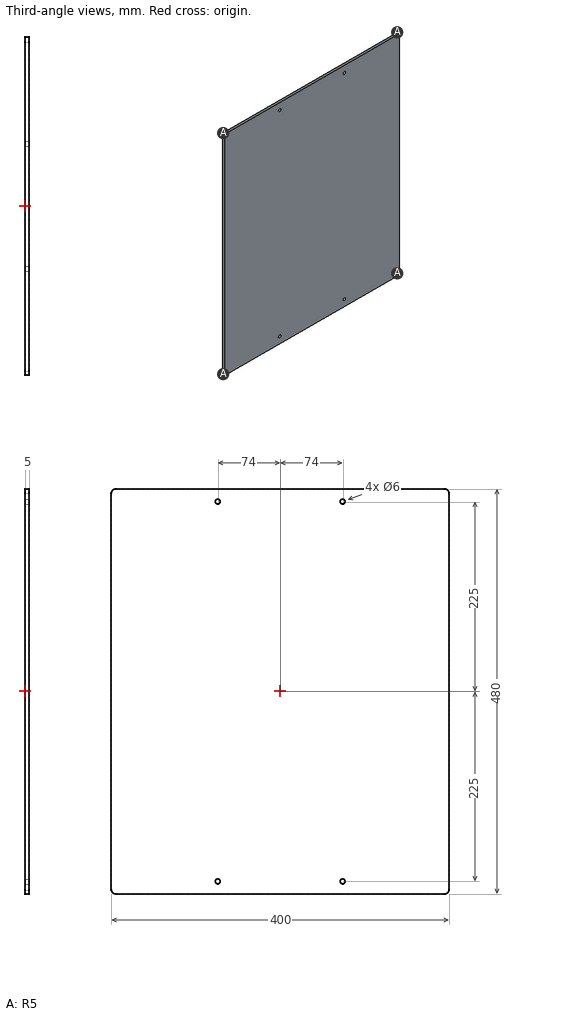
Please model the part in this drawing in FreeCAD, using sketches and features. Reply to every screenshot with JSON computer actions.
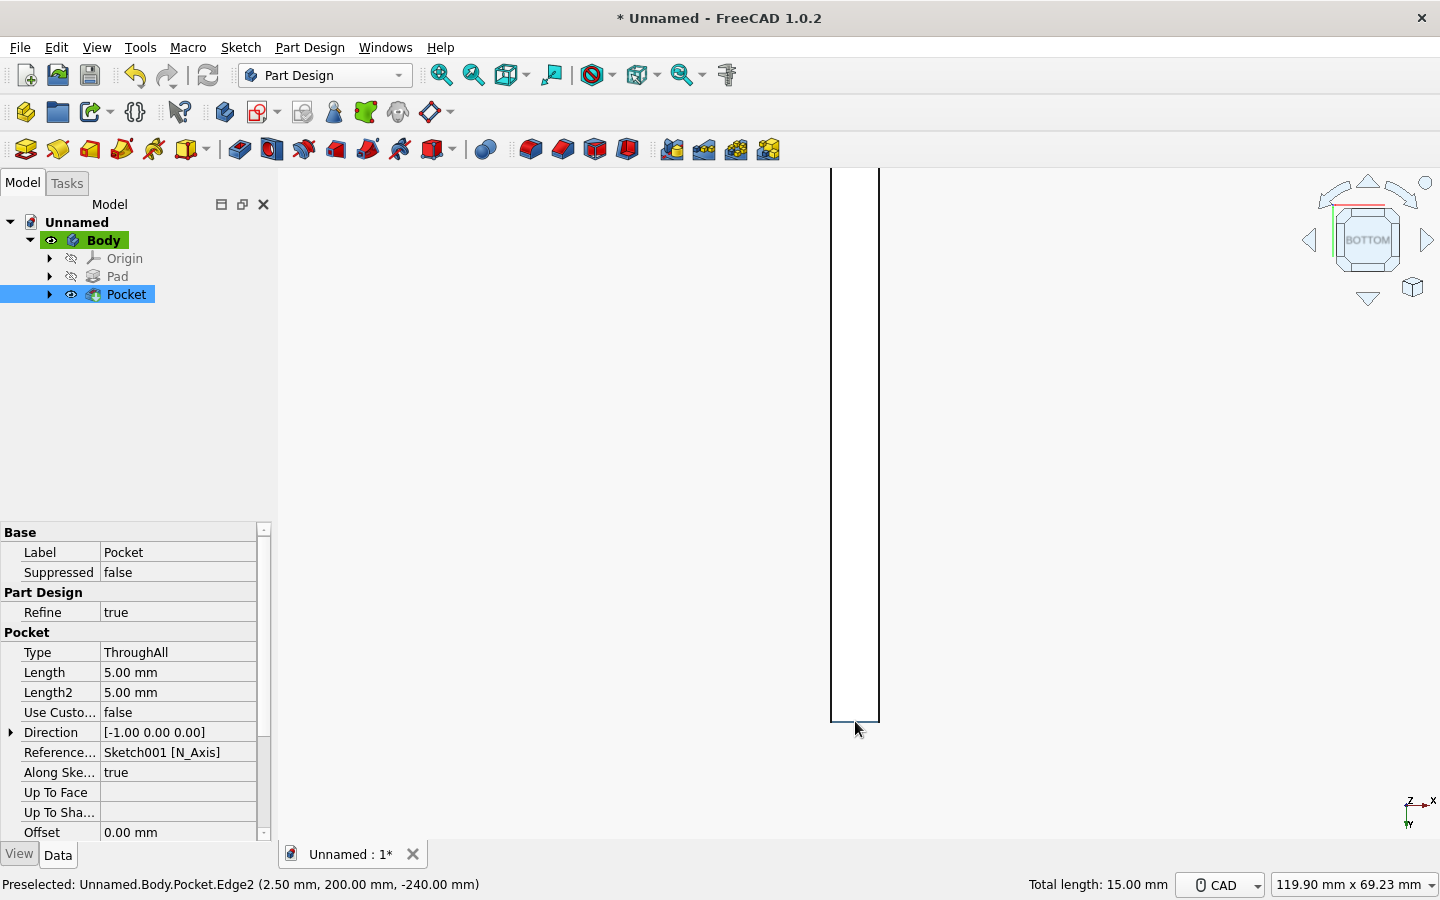
{"action": "key", "text": "v f"}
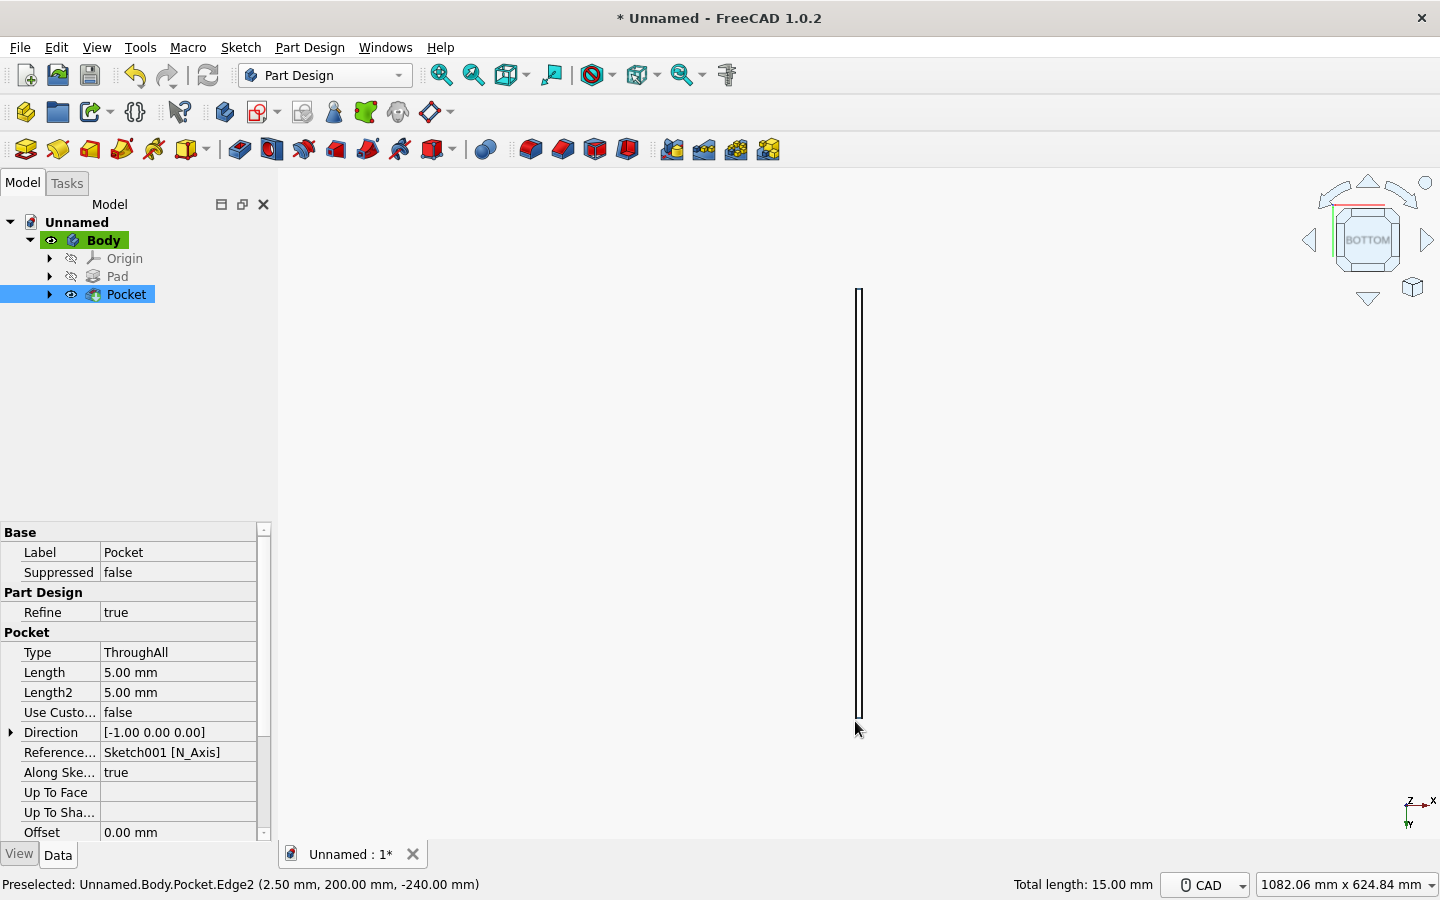
{"action": "key", "text": "4"}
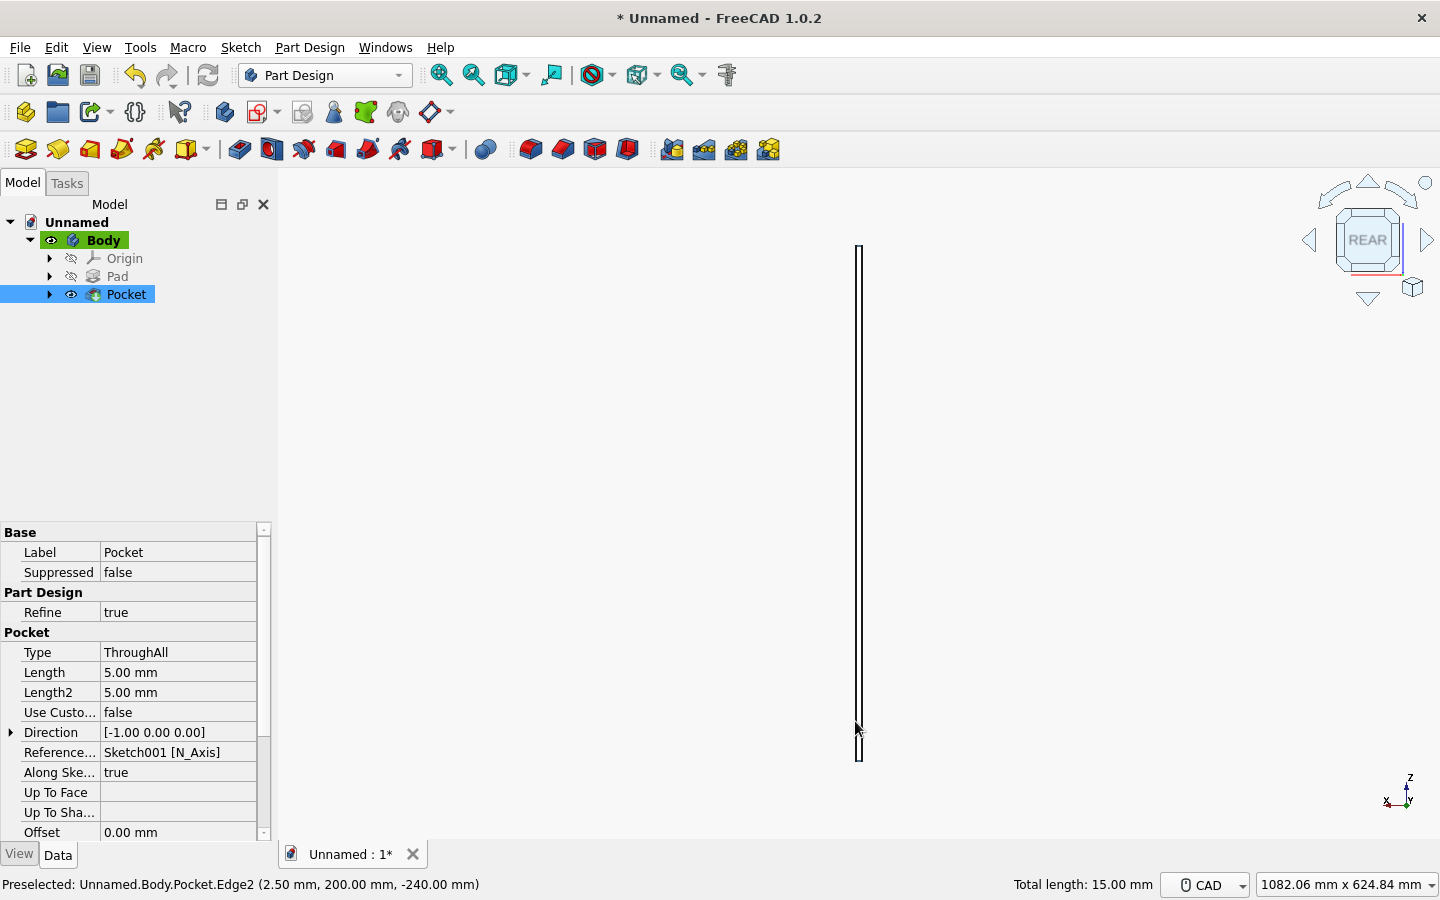
{"action": "scroll", "coordinate": [859, 245], "scroll_direction": "up", "scroll_amount": 11}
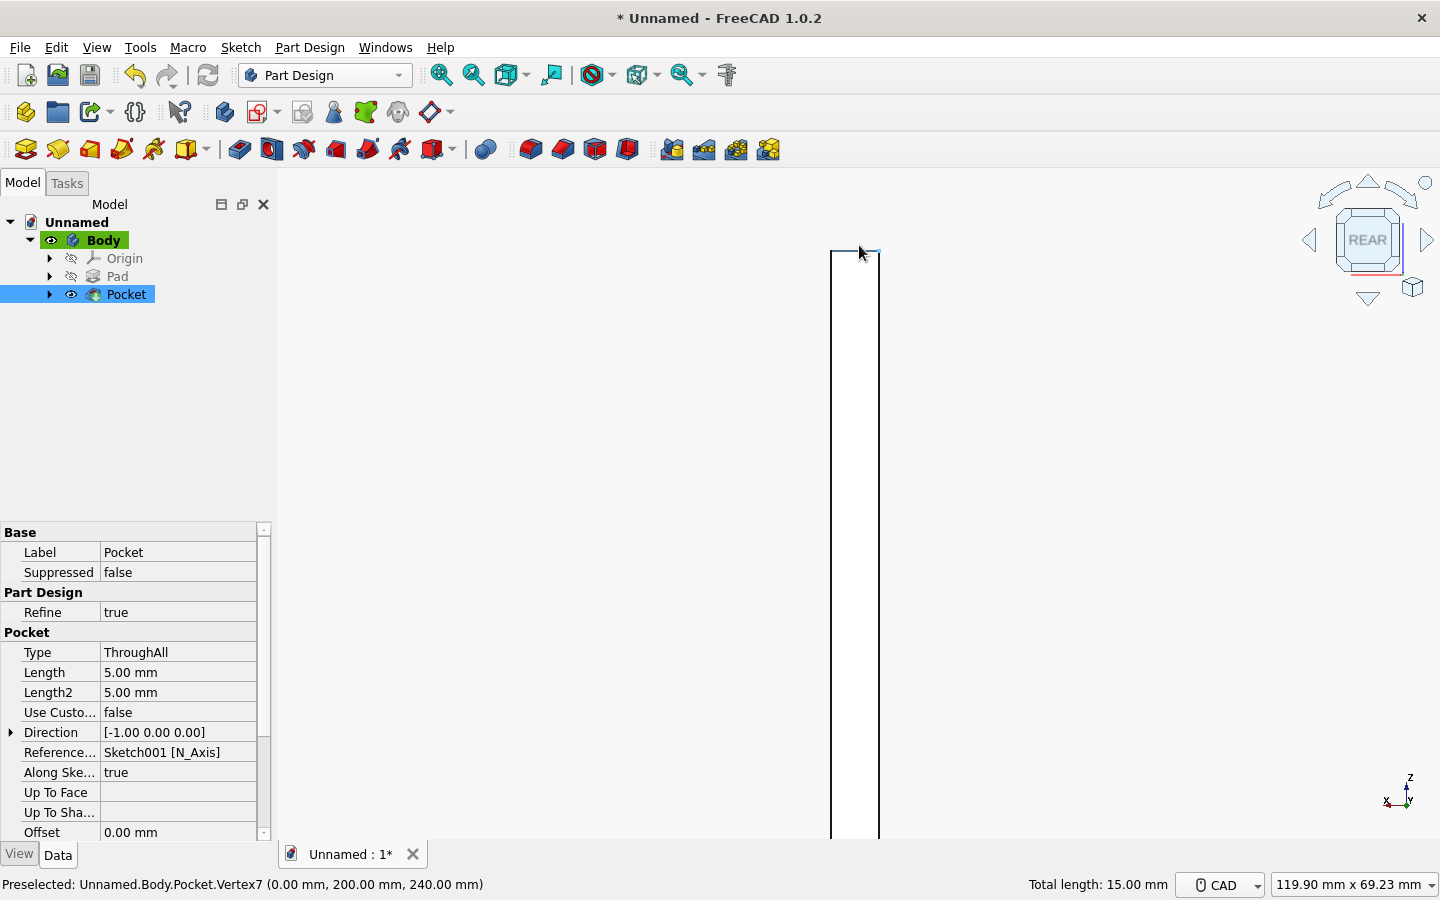
{"action": "left_click", "coordinate": [442, 76]}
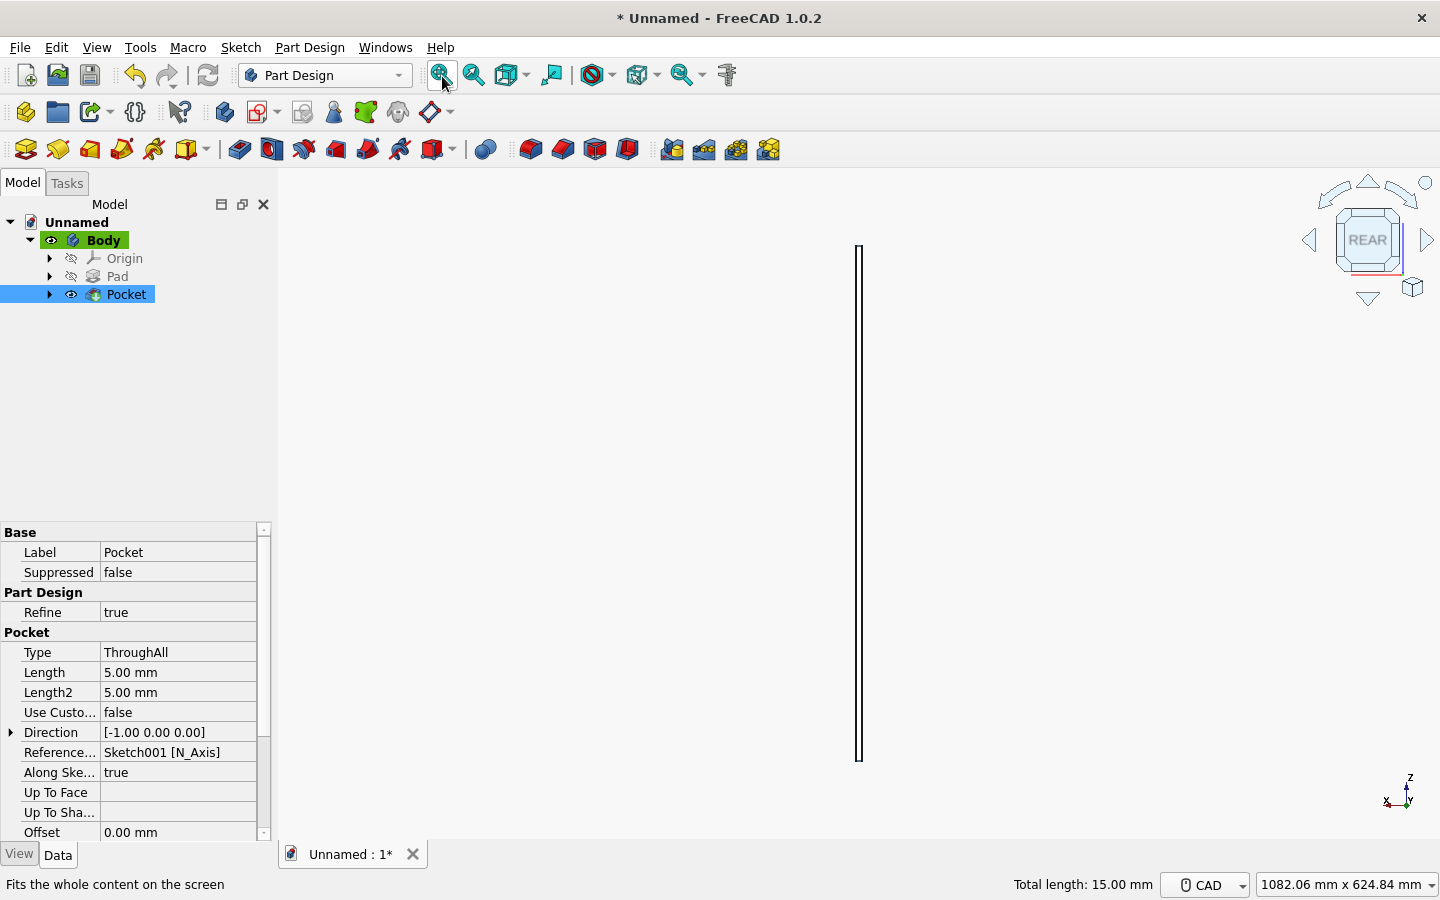
{"action": "key", "text": "6"}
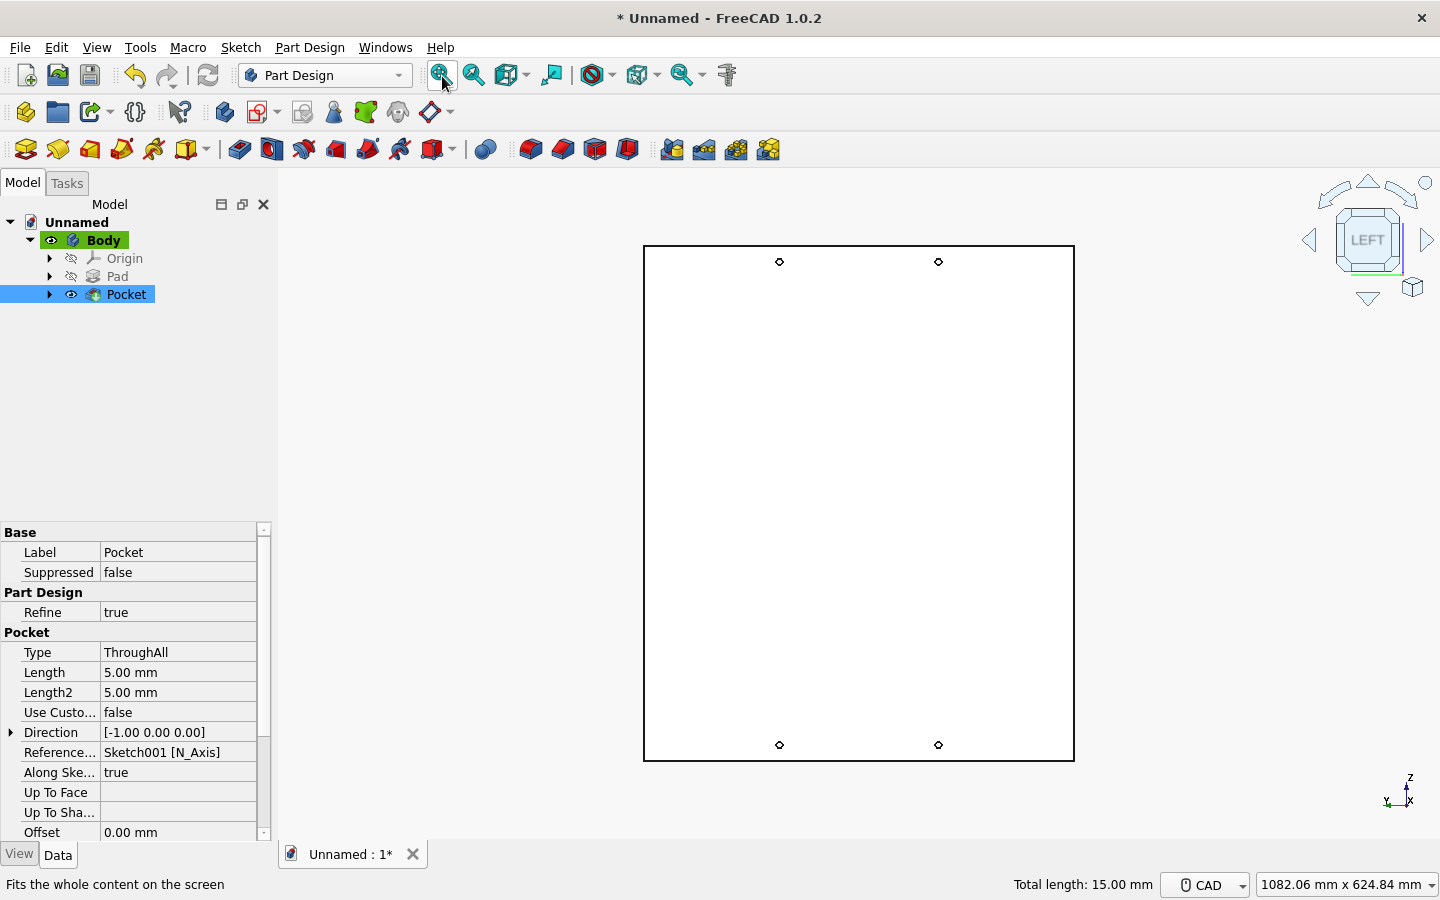
{"action": "scroll", "coordinate": [1074, 245], "scroll_direction": "up", "scroll_amount": 11}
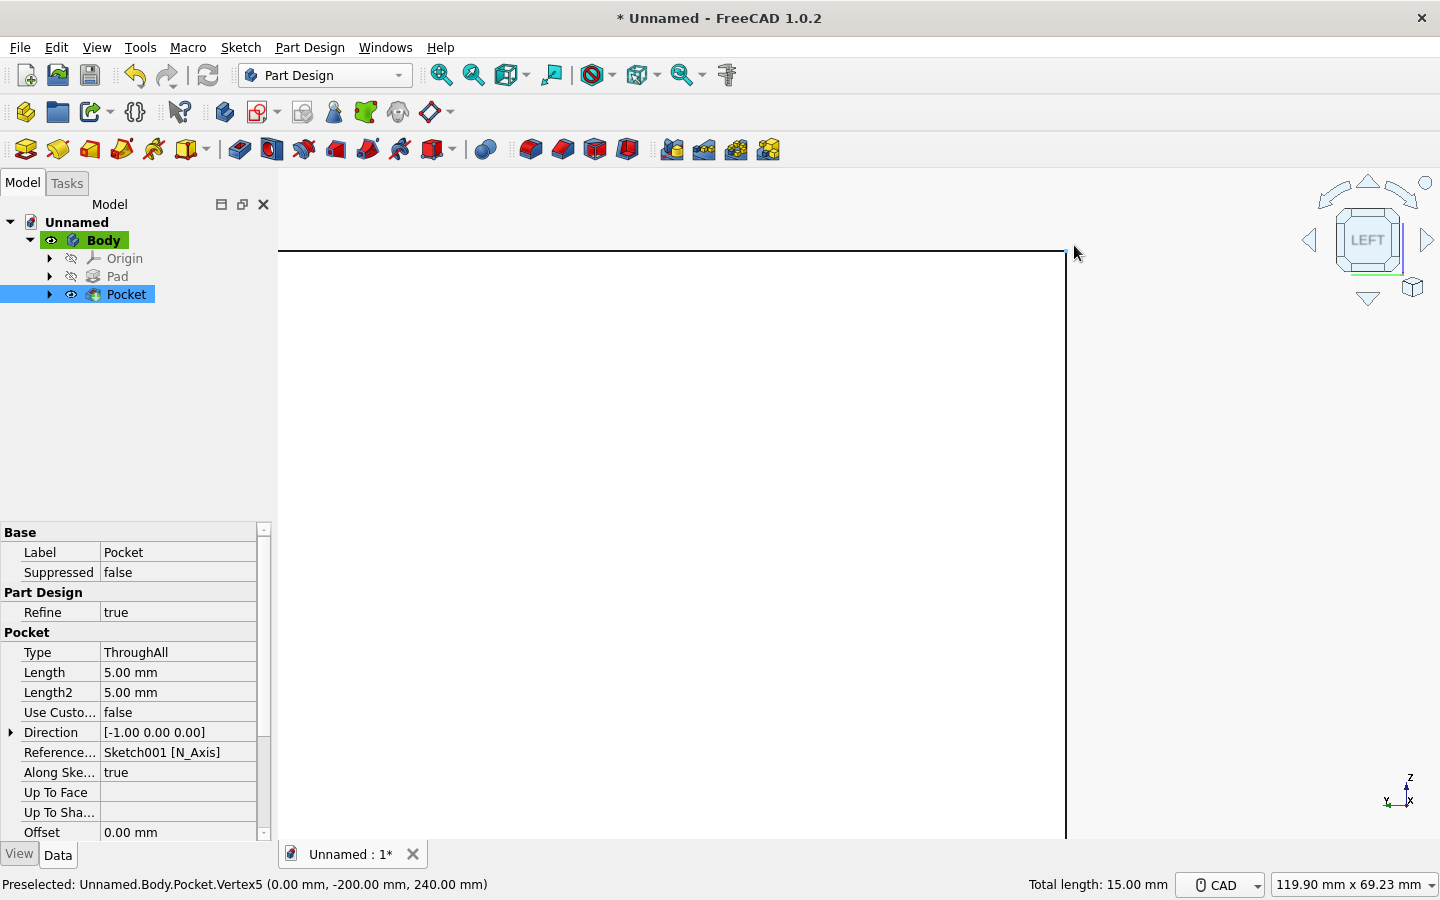
{"action": "left_click", "coordinate": [442, 76]}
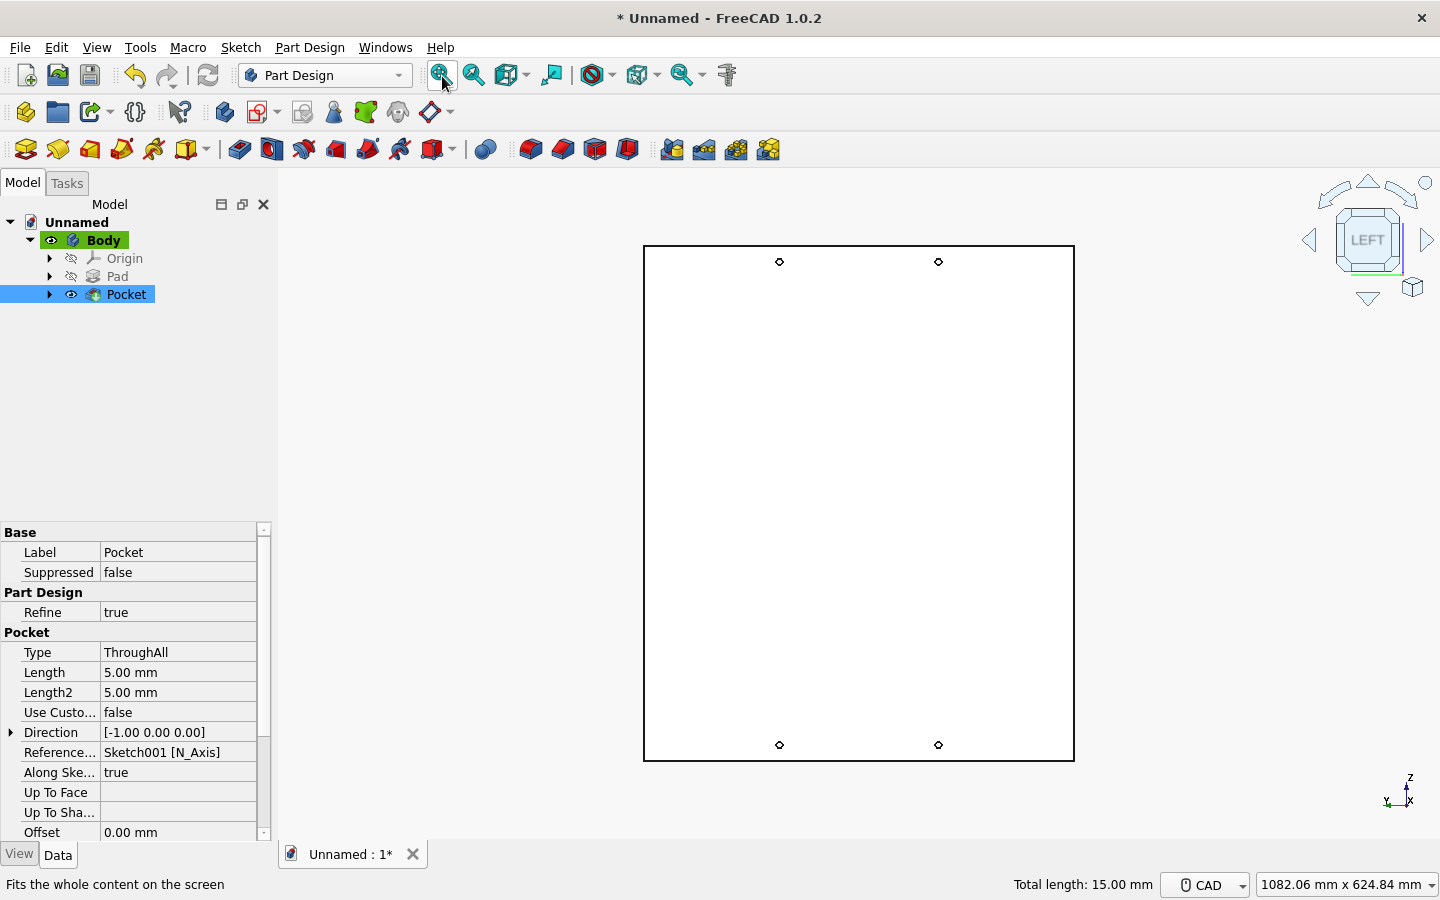
{"action": "key", "text": "v 3"}